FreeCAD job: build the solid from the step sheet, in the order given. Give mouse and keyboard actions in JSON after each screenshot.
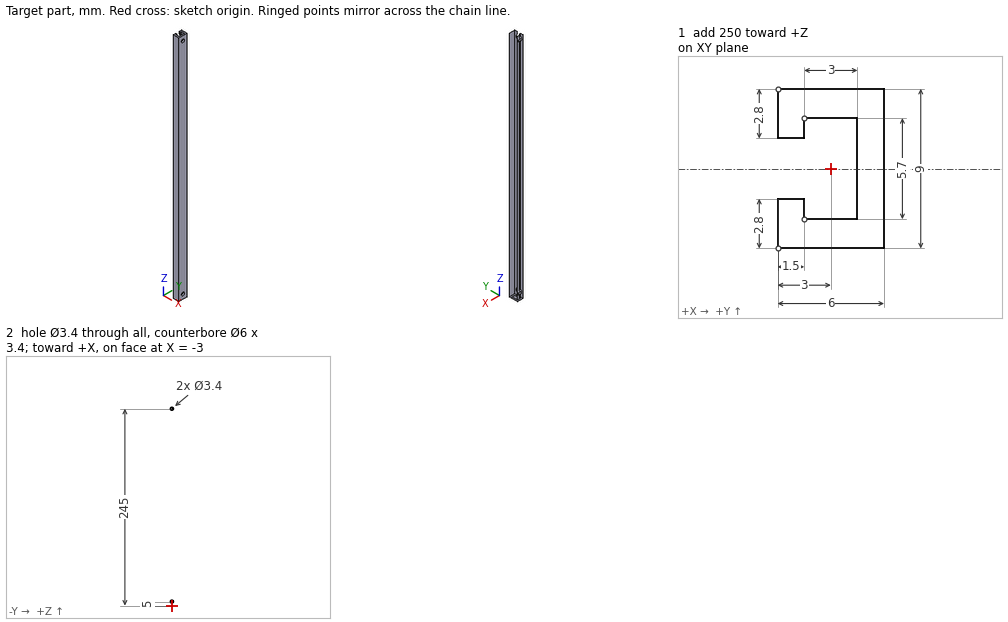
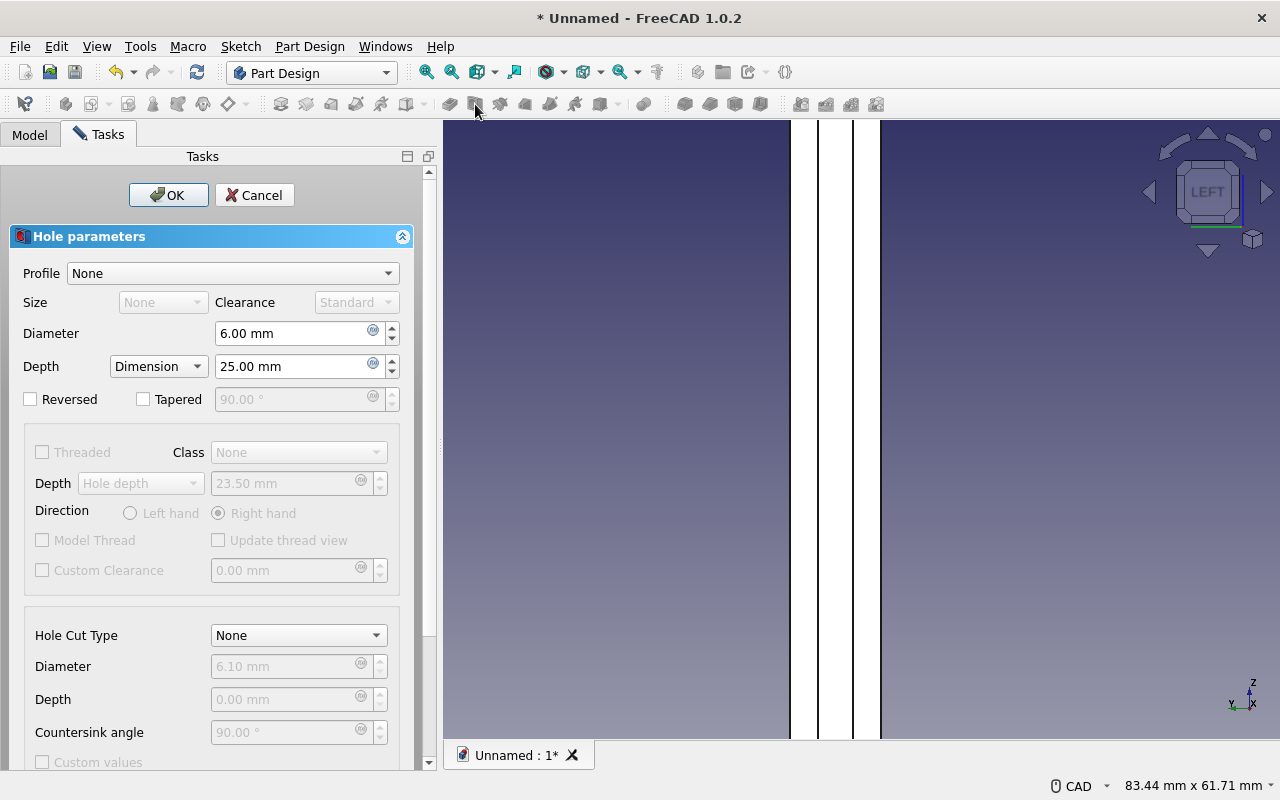
{"action": "triple_click", "coordinate": [300, 334]}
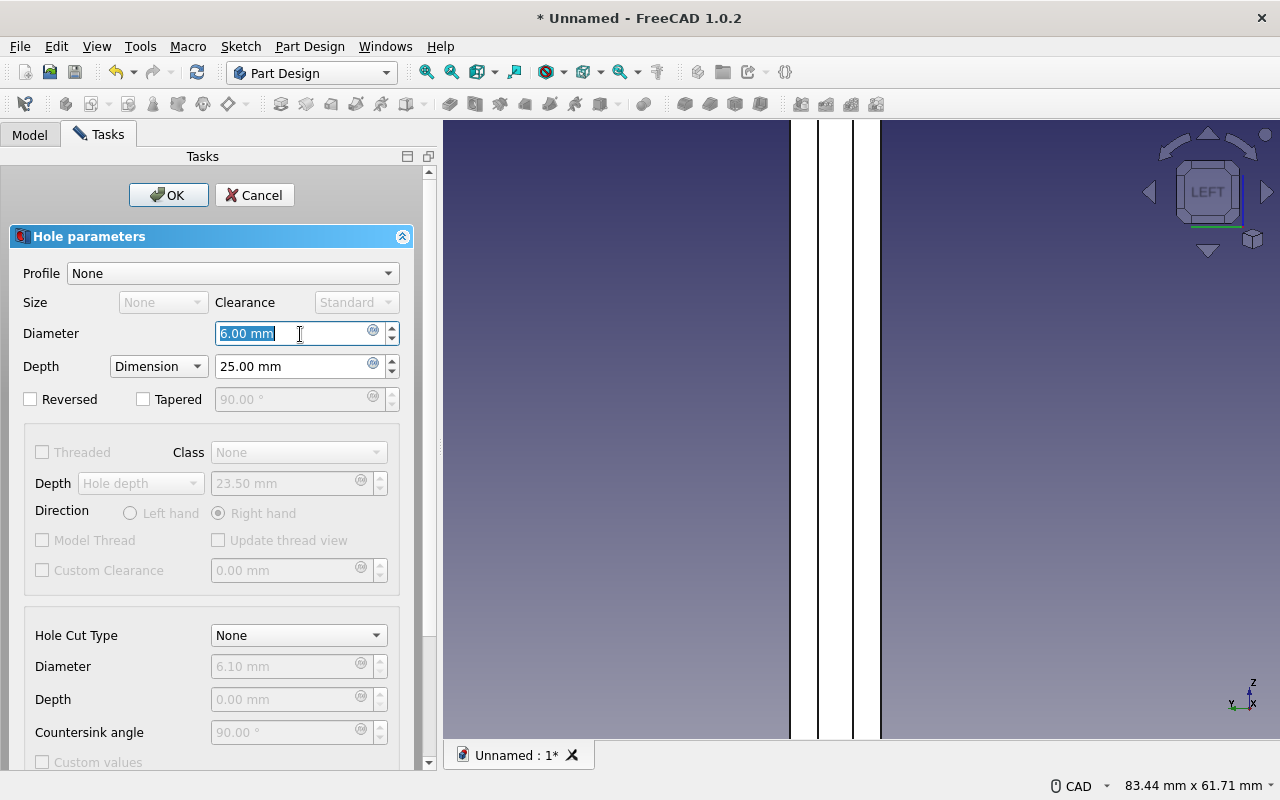
{"action": "type", "text": "3.4"}
{"action": "key", "text": "Tab"}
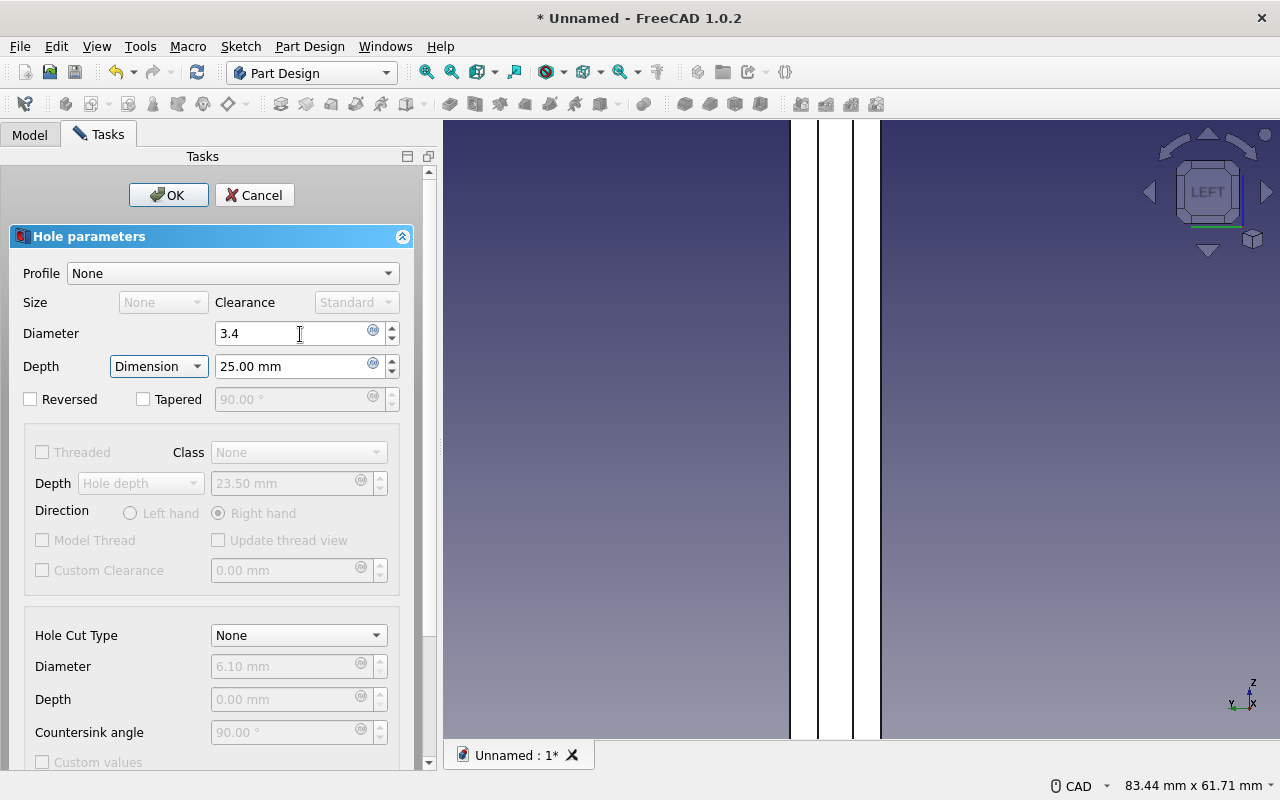
{"action": "left_click", "coordinate": [160, 366]}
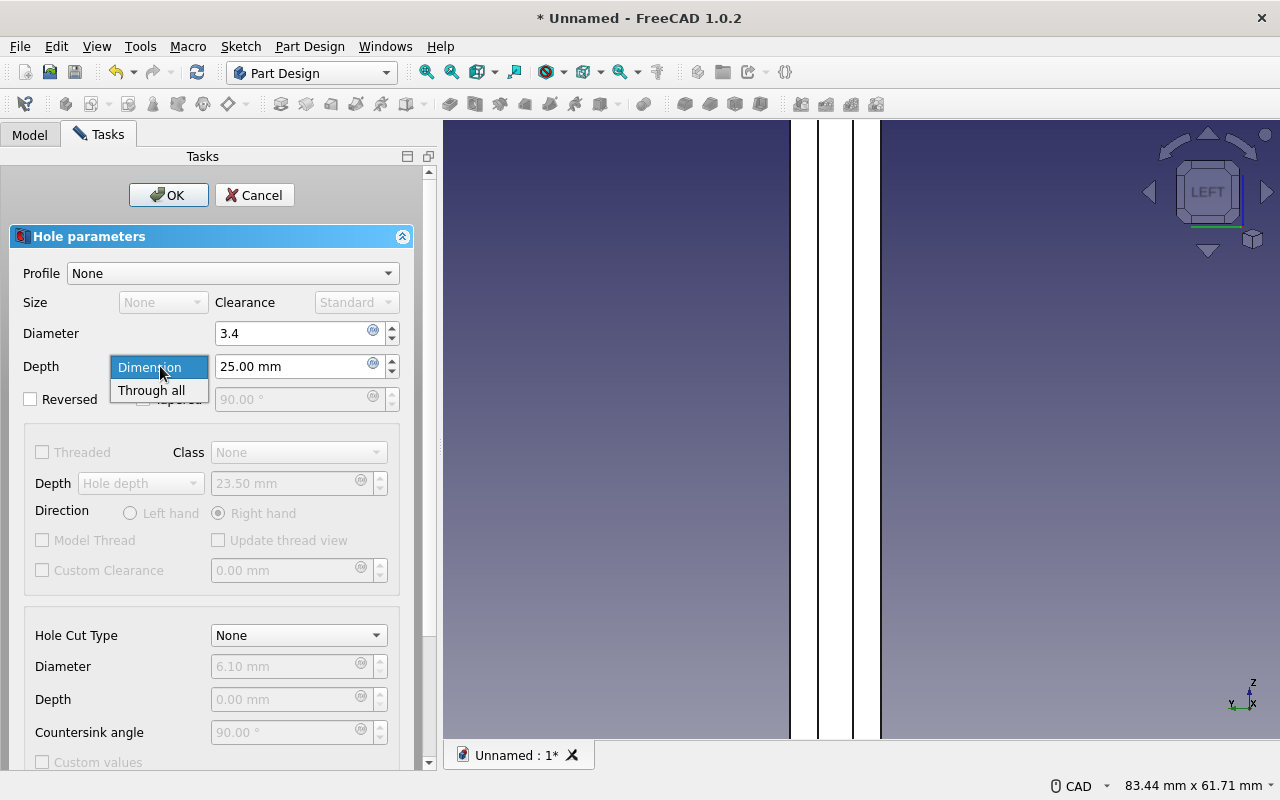
{"action": "left_click", "coordinate": [158, 390]}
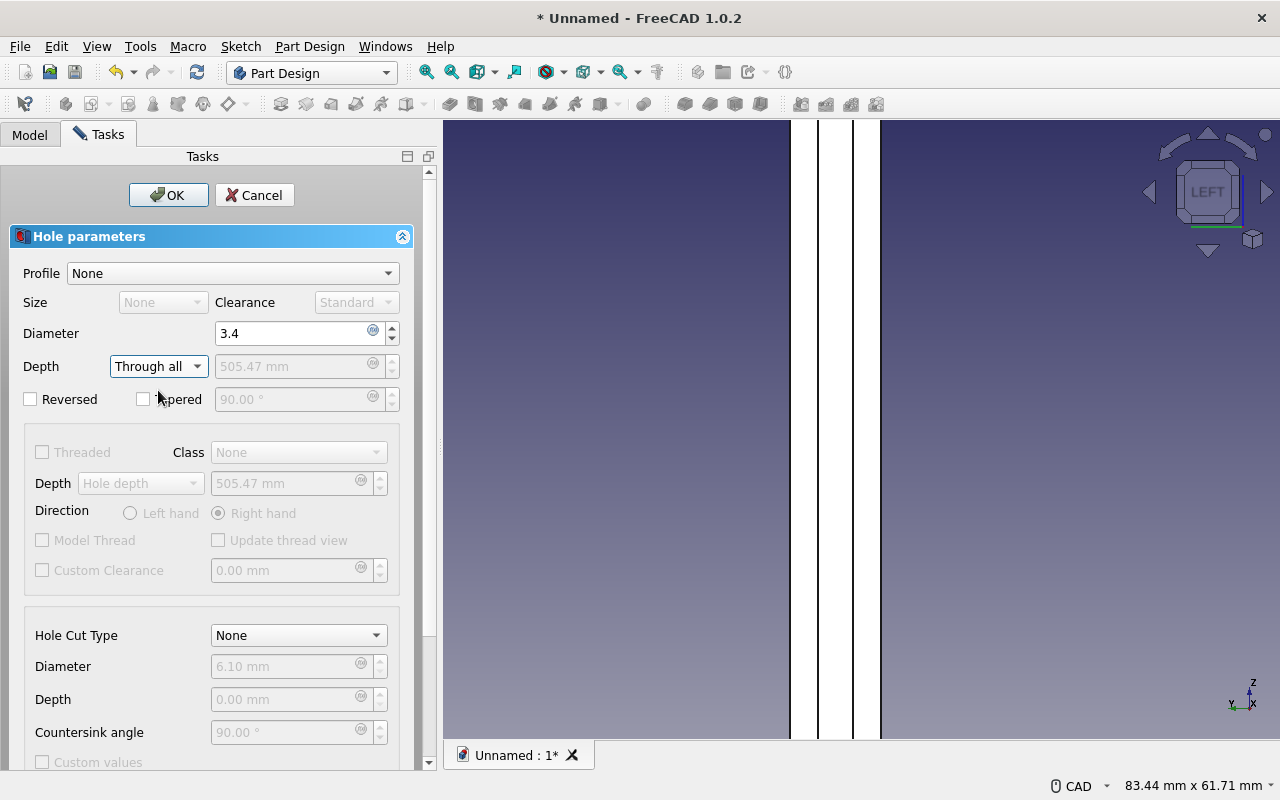
{"action": "left_click", "coordinate": [300, 636]}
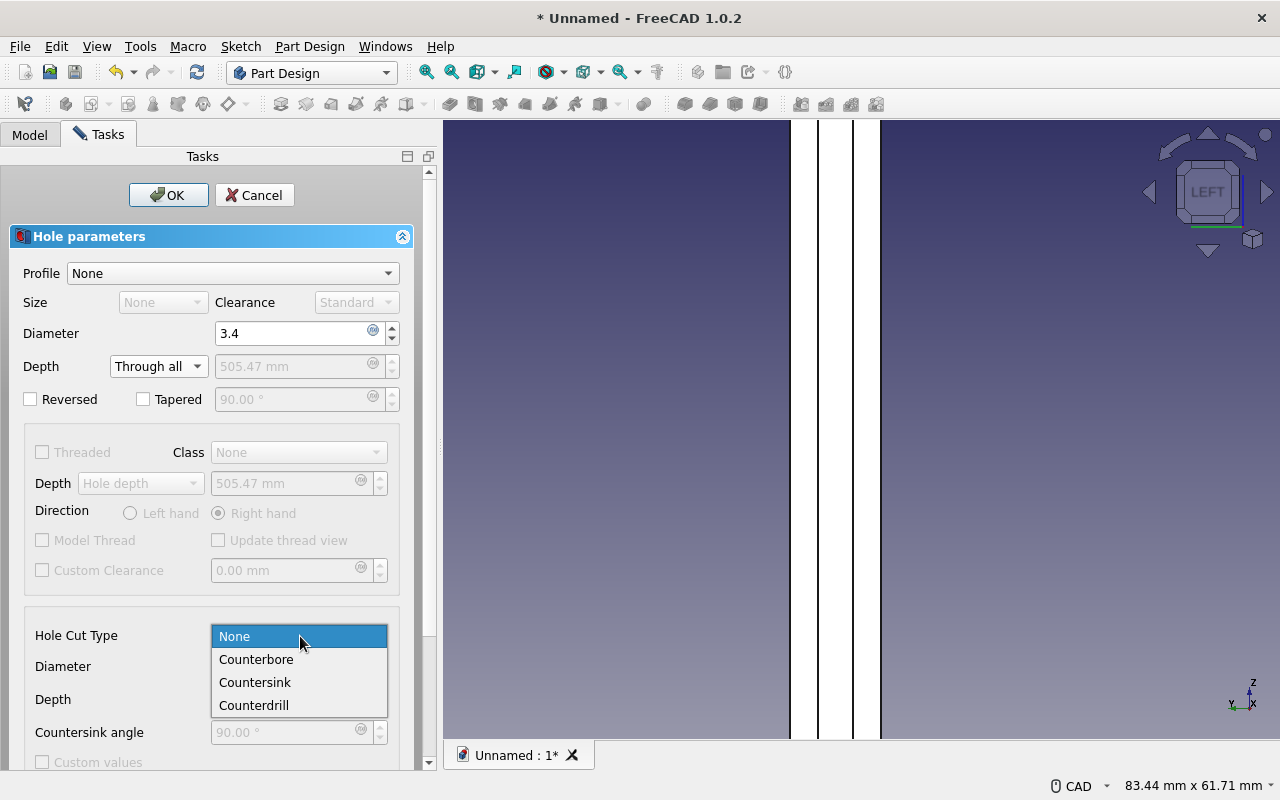
{"action": "left_click", "coordinate": [298, 660]}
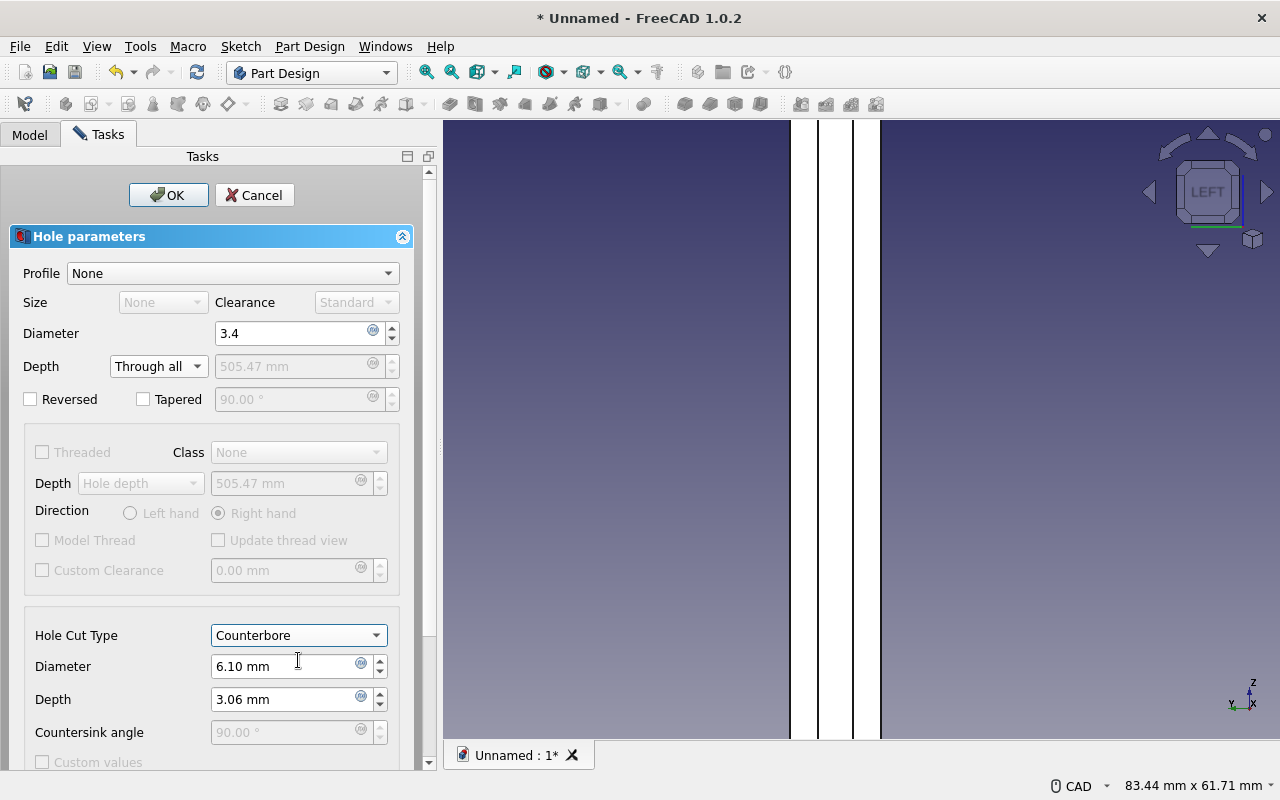
{"action": "triple_click", "coordinate": [292, 666]}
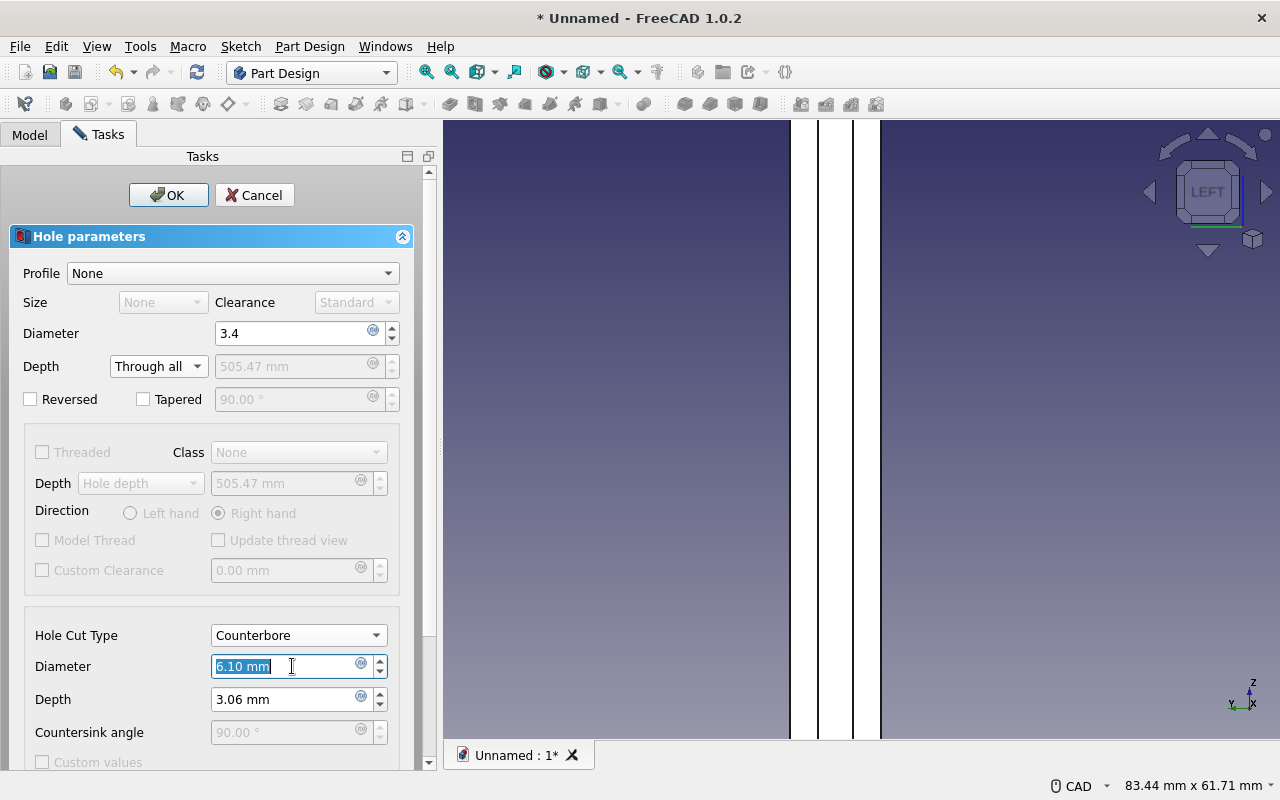
{"action": "type", "text": "6"}
{"action": "key", "text": "Tab"}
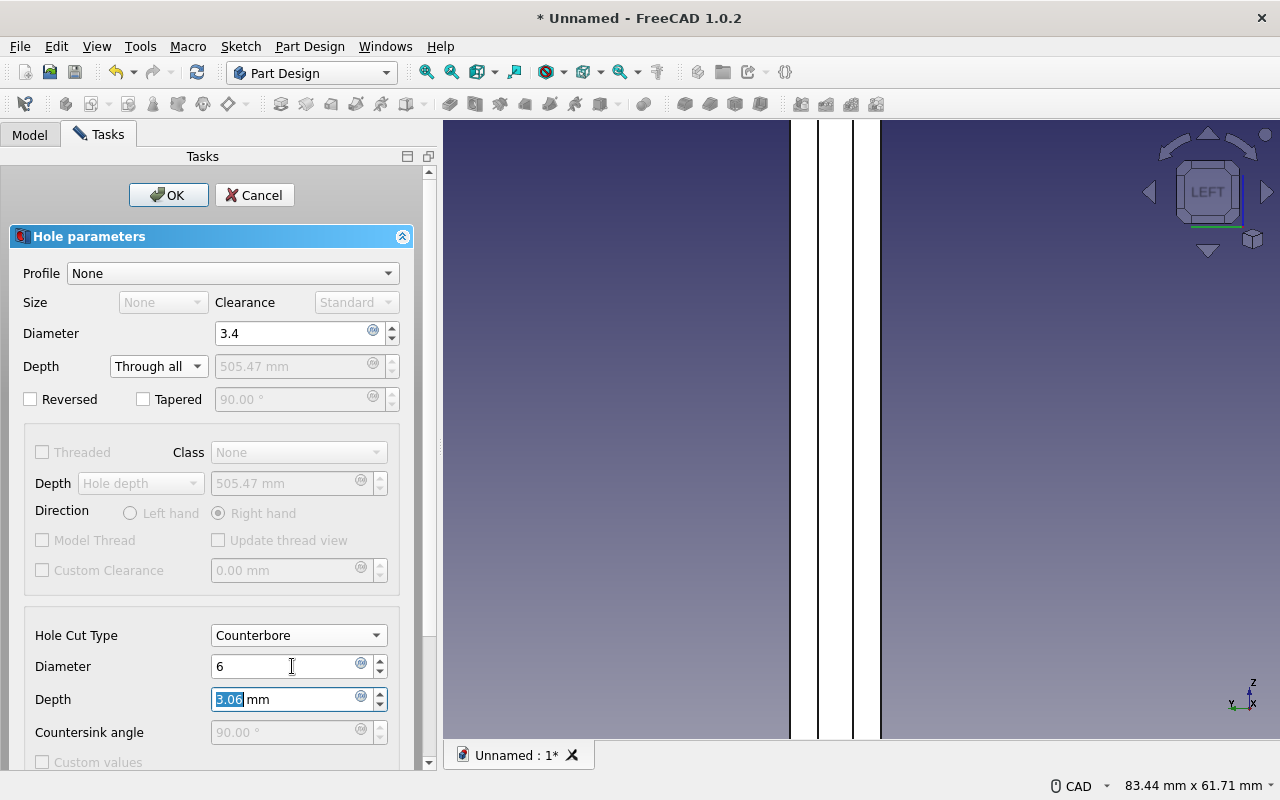
{"action": "type", "text": "3.4"}
{"action": "key", "text": "Tab"}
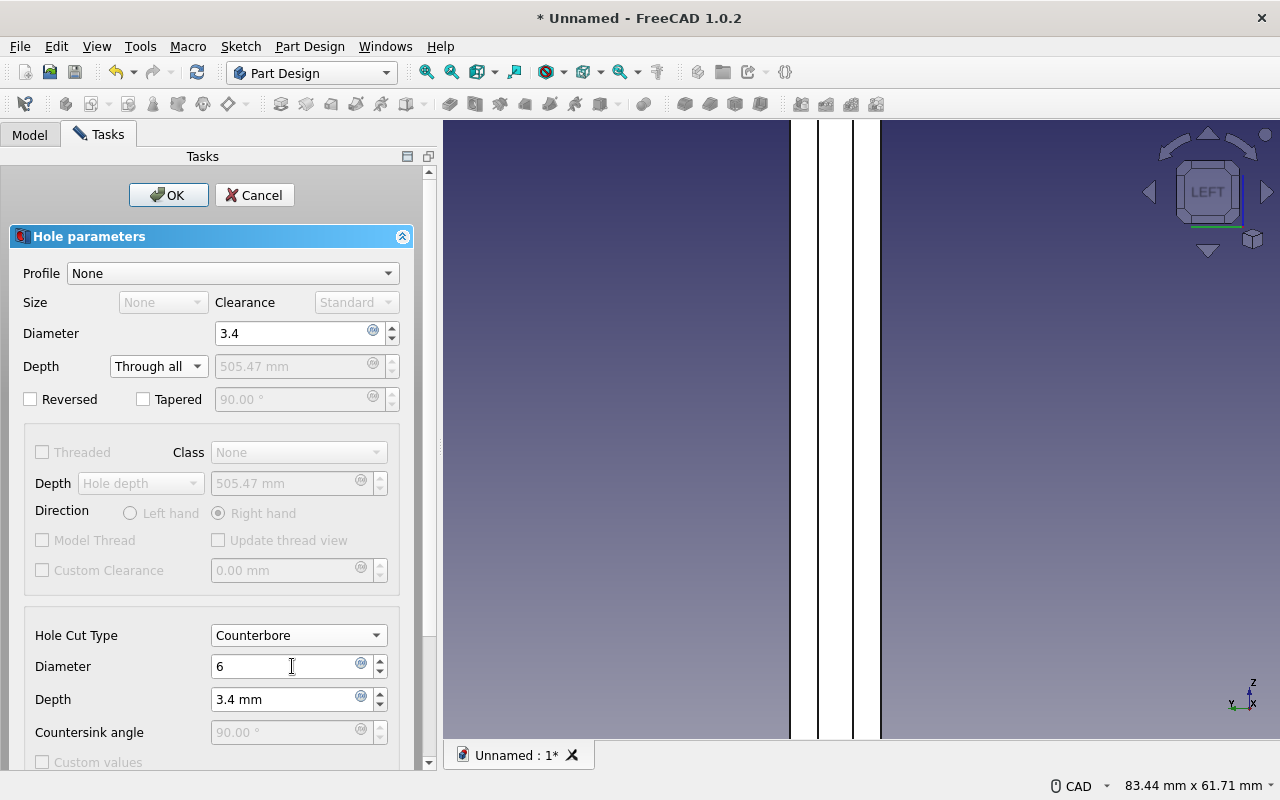
{"action": "left_click", "coordinate": [169, 195]}